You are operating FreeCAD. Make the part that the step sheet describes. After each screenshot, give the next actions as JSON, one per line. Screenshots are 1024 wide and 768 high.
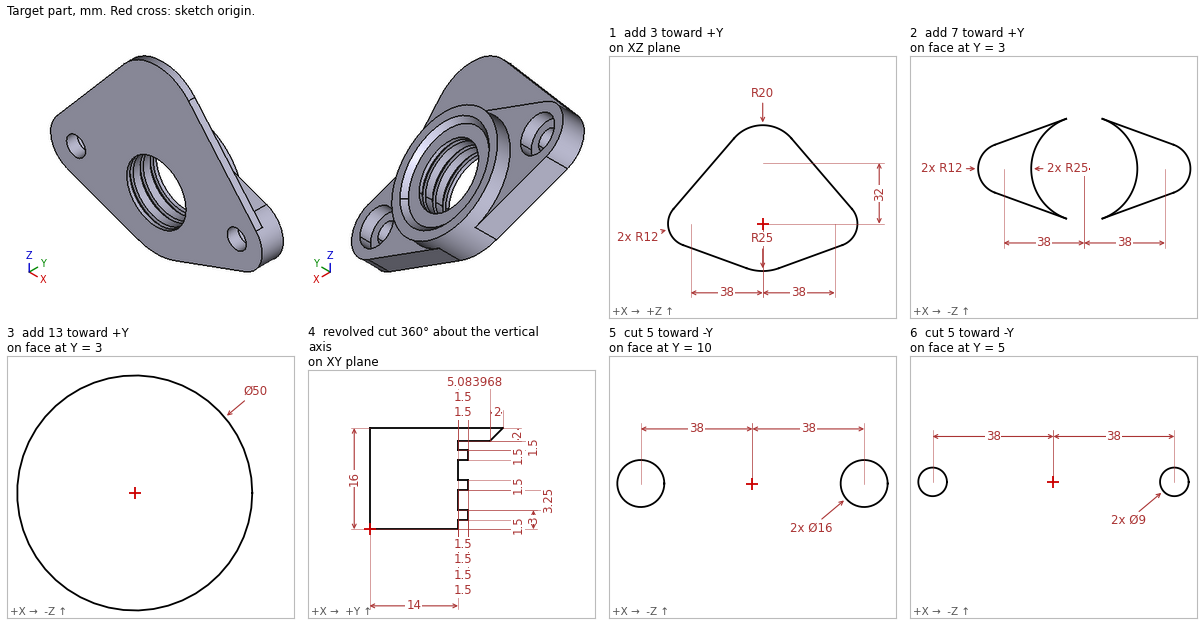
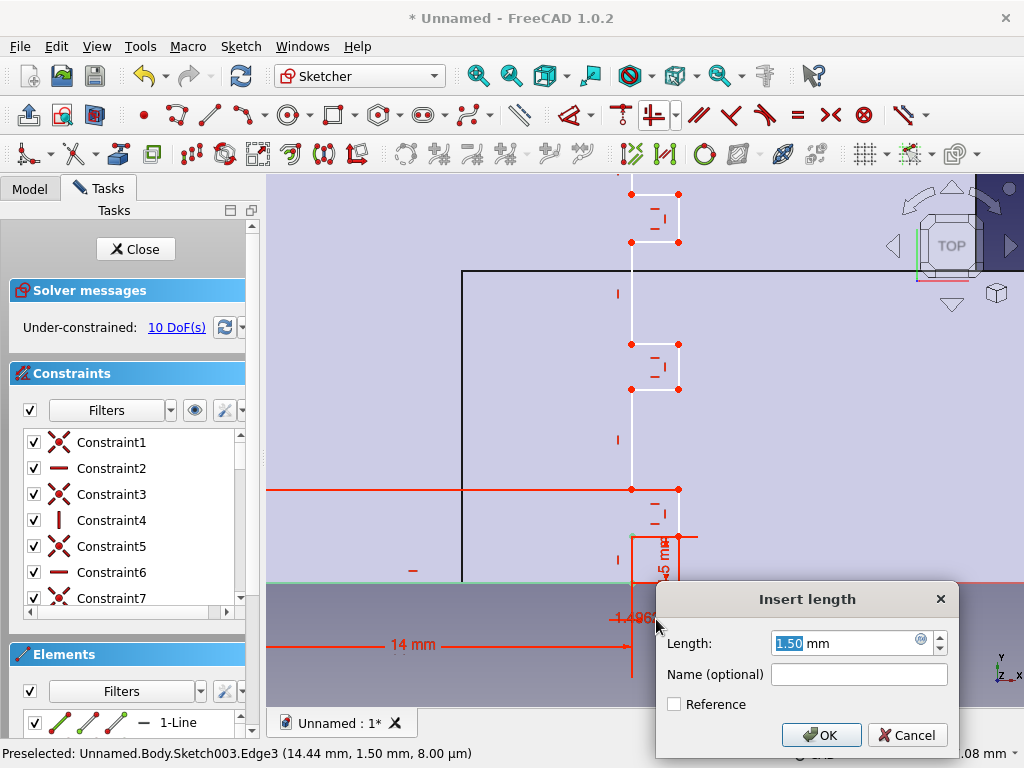
{"action": "type", "text": "1.5"}
{"action": "key", "text": "Return"}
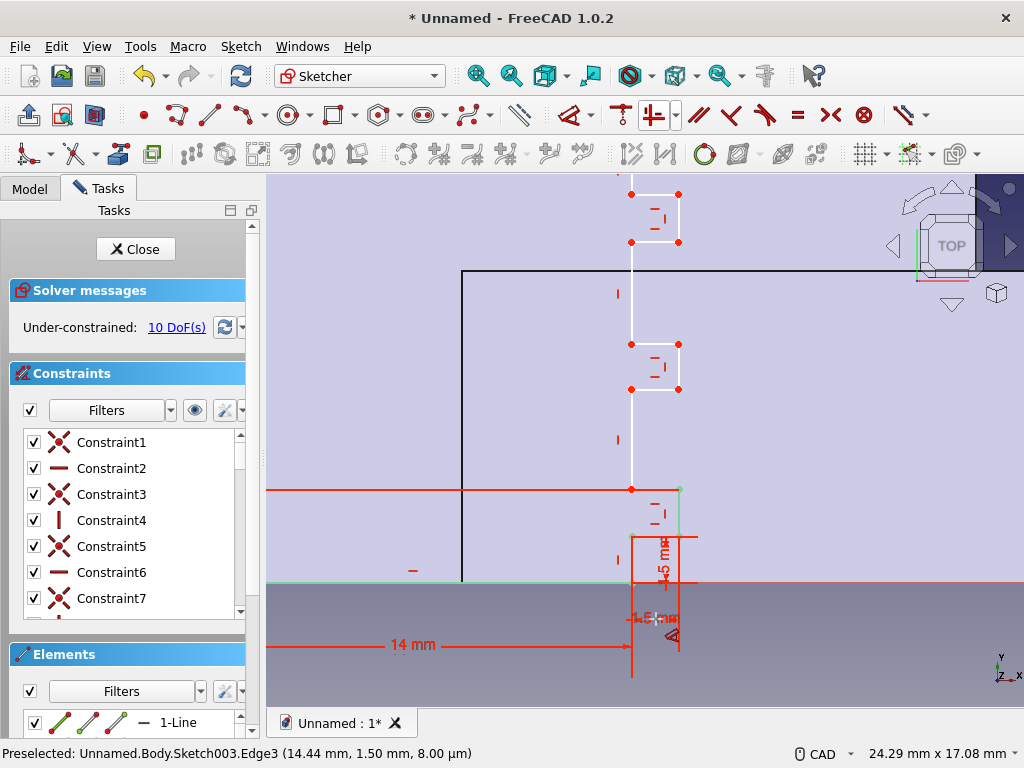
{"action": "left_click", "coordinate": [665, 490]}
{"action": "left_click", "coordinate": [655, 456]}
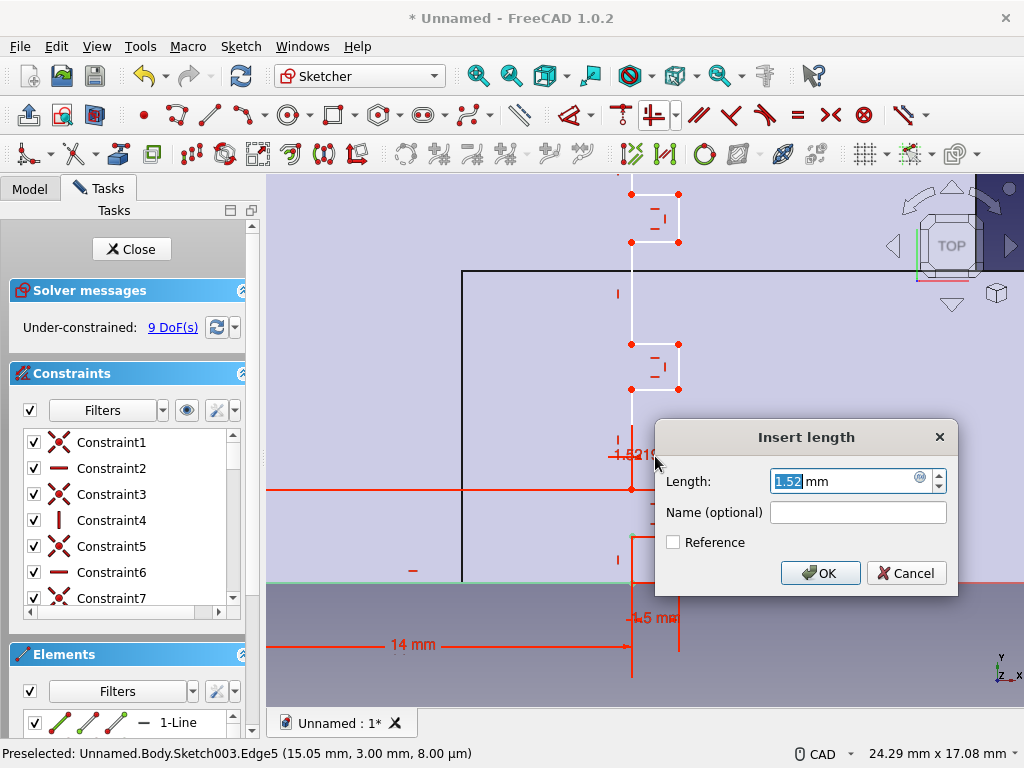
{"action": "type", "text": "1.5"}
{"action": "key", "text": "Return"}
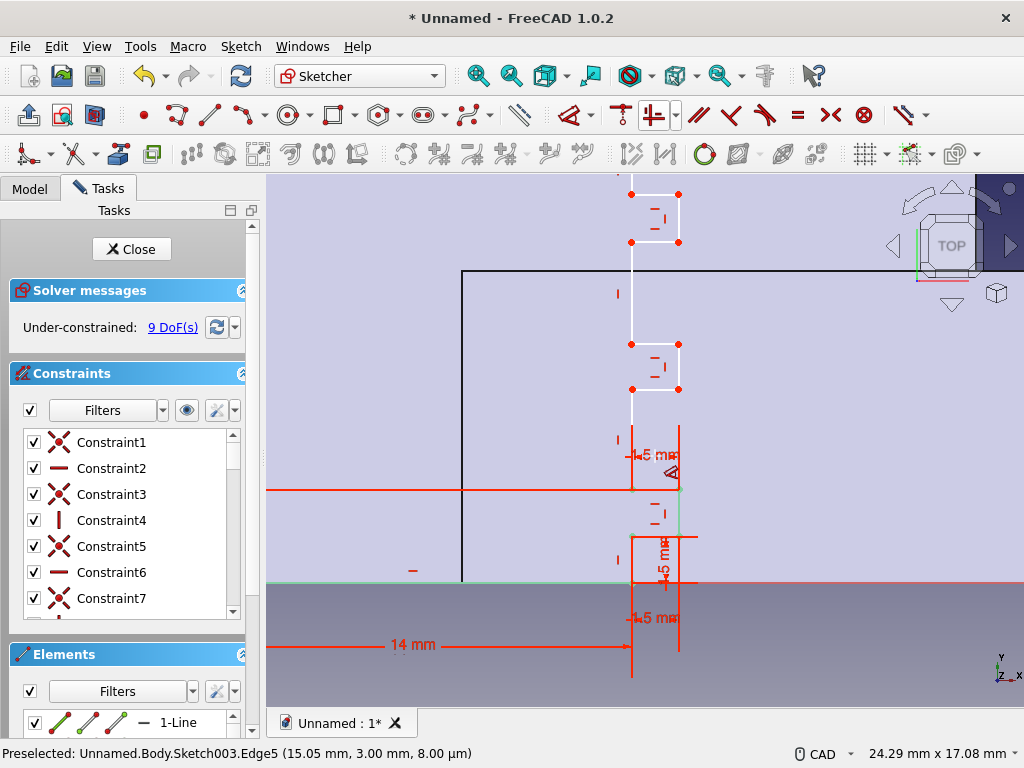
{"action": "left_click", "coordinate": [646, 390]}
{"action": "left_click", "coordinate": [656, 424]}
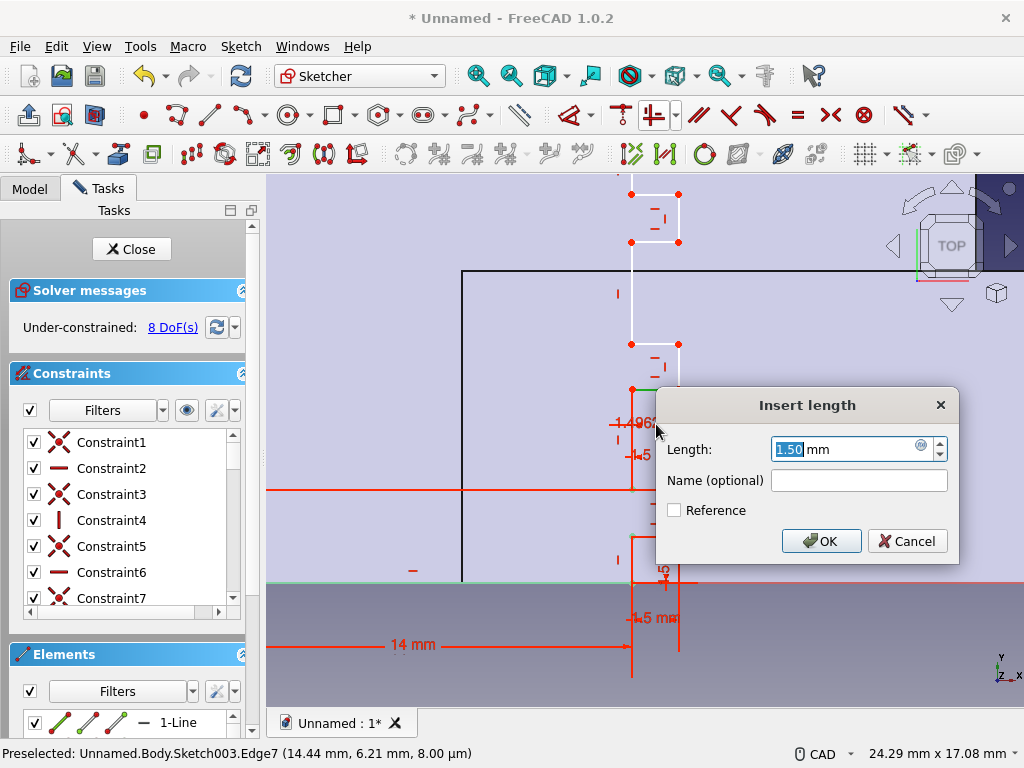
{"action": "type", "text": "1.5"}
{"action": "key", "text": "Return"}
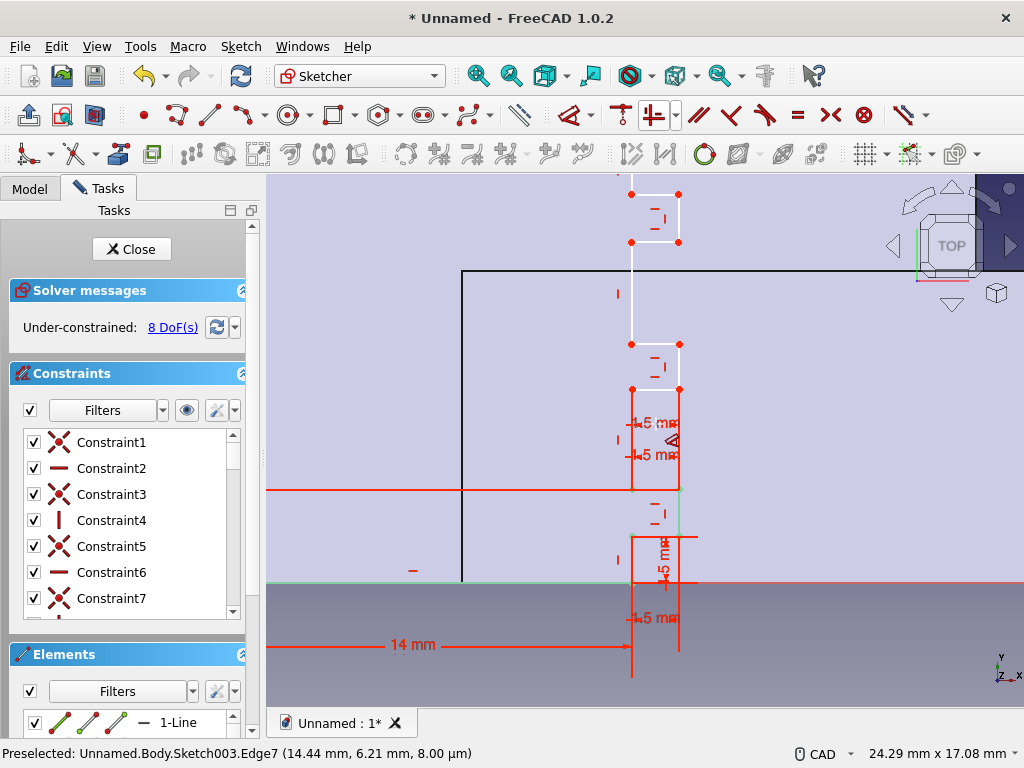
{"action": "left_click", "coordinate": [679, 376]}
{"action": "left_click", "coordinate": [713, 367]}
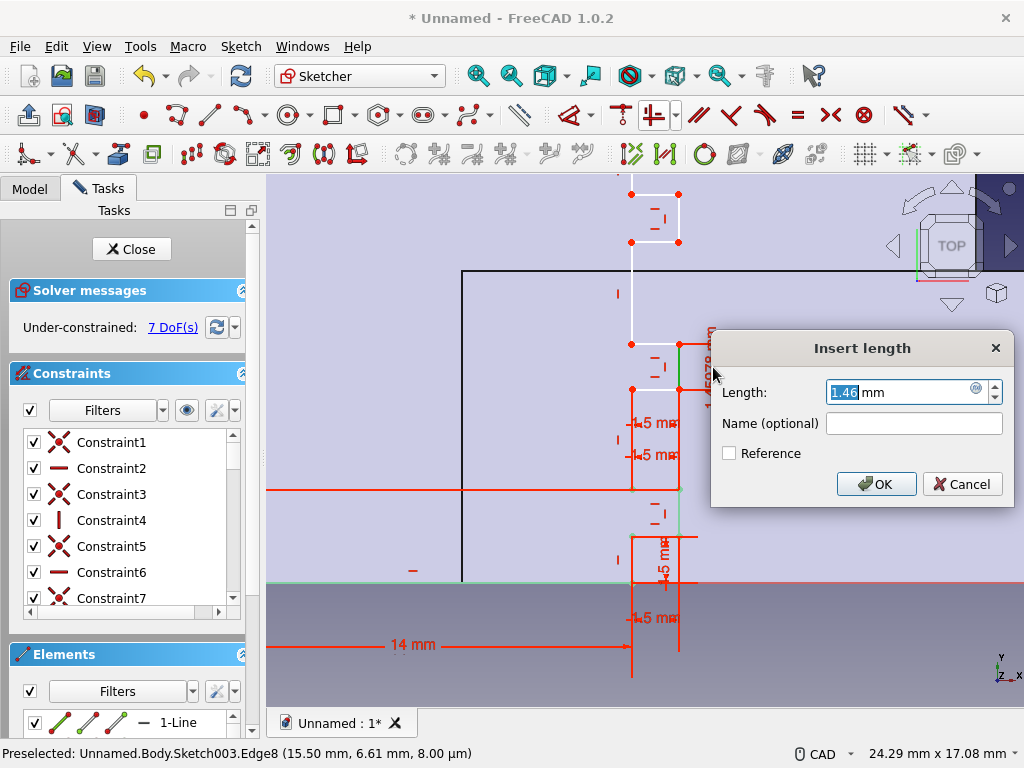
{"action": "type", "text": "1.5"}
{"action": "key", "text": "Return"}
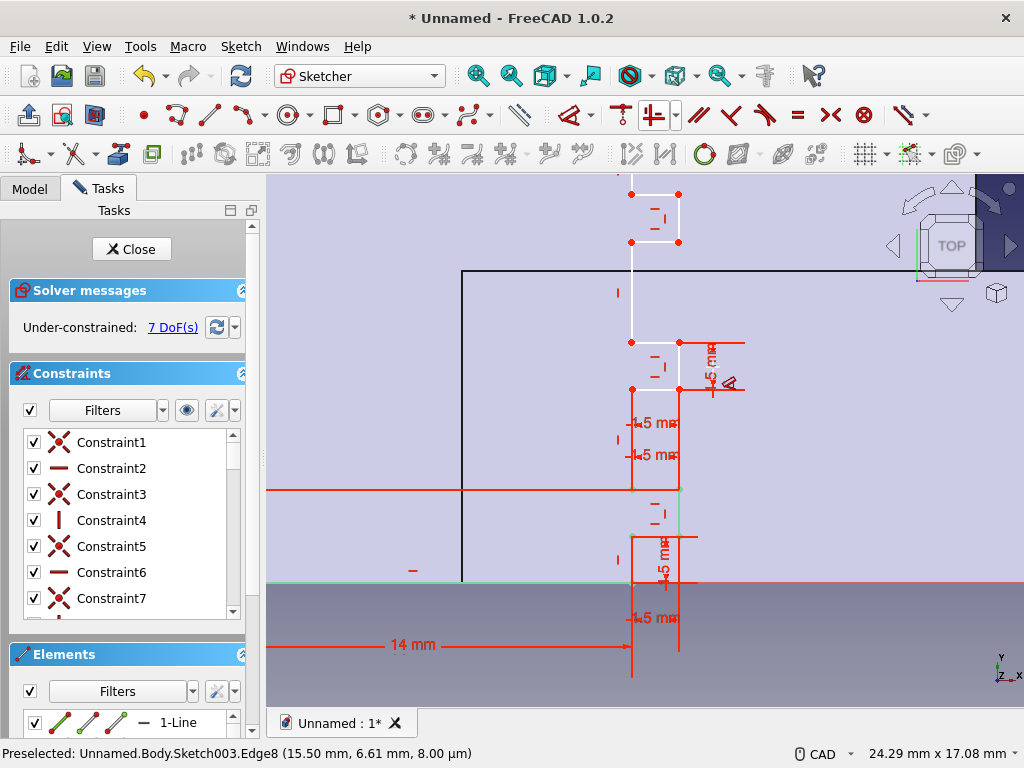
{"action": "left_click", "coordinate": [665, 343]}
{"action": "left_click", "coordinate": [655, 309]}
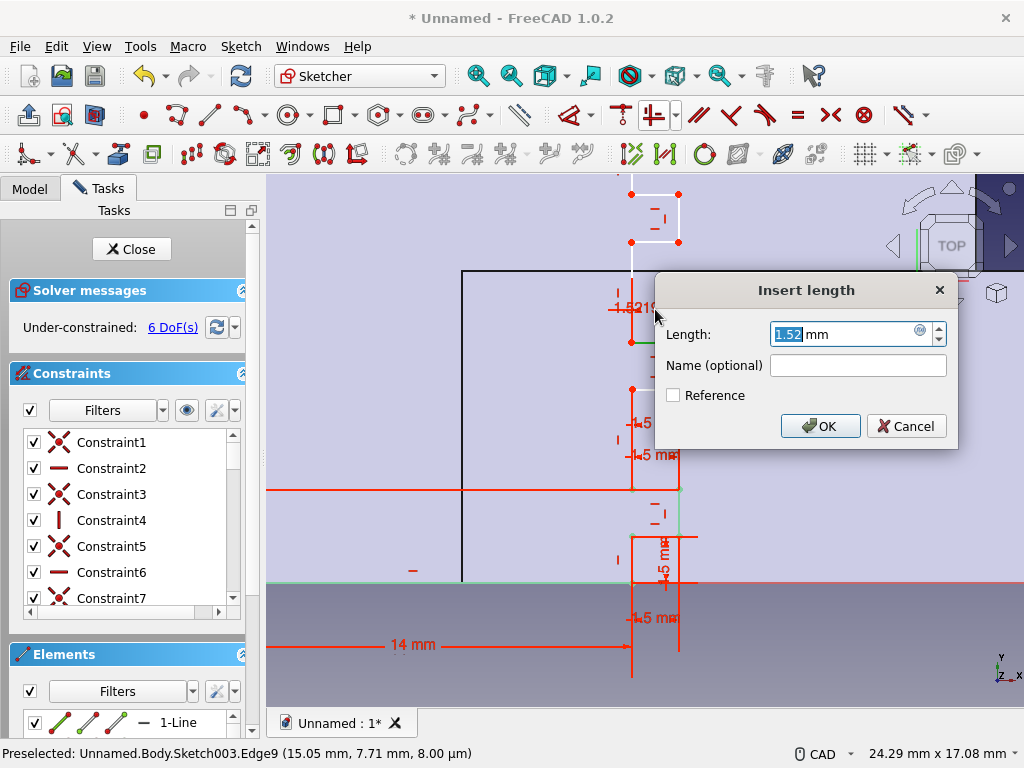
{"action": "type", "text": "1.5"}
{"action": "key", "text": "Return"}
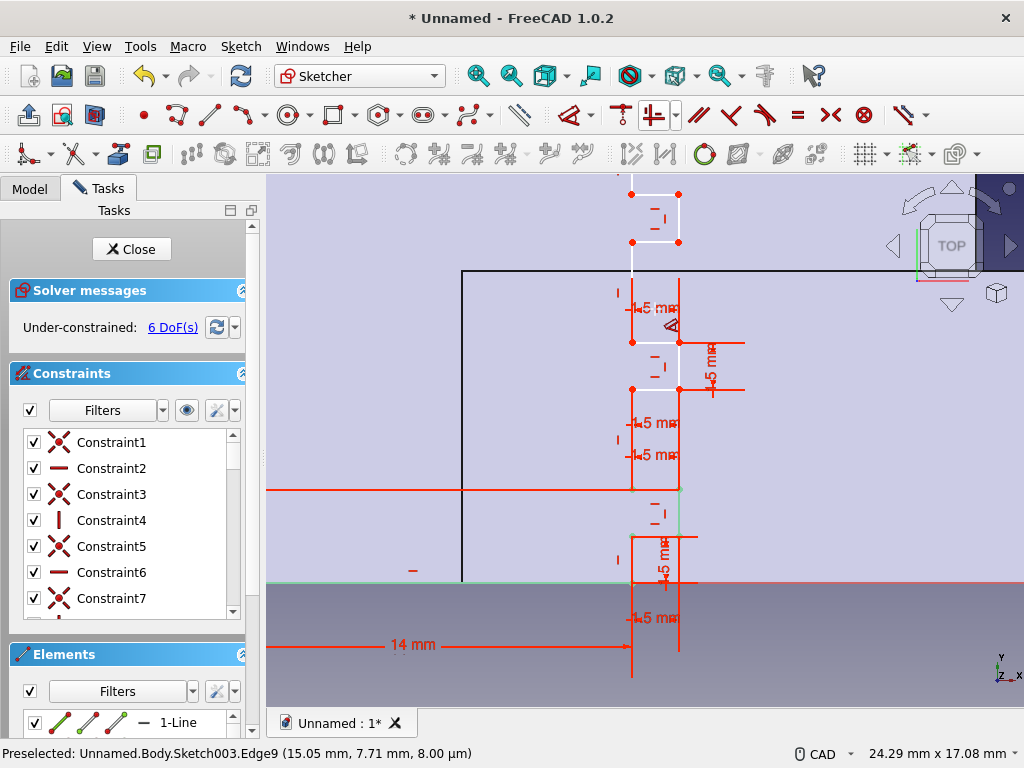
{"action": "left_click", "coordinate": [646, 242]}
{"action": "left_click", "coordinate": [656, 208]}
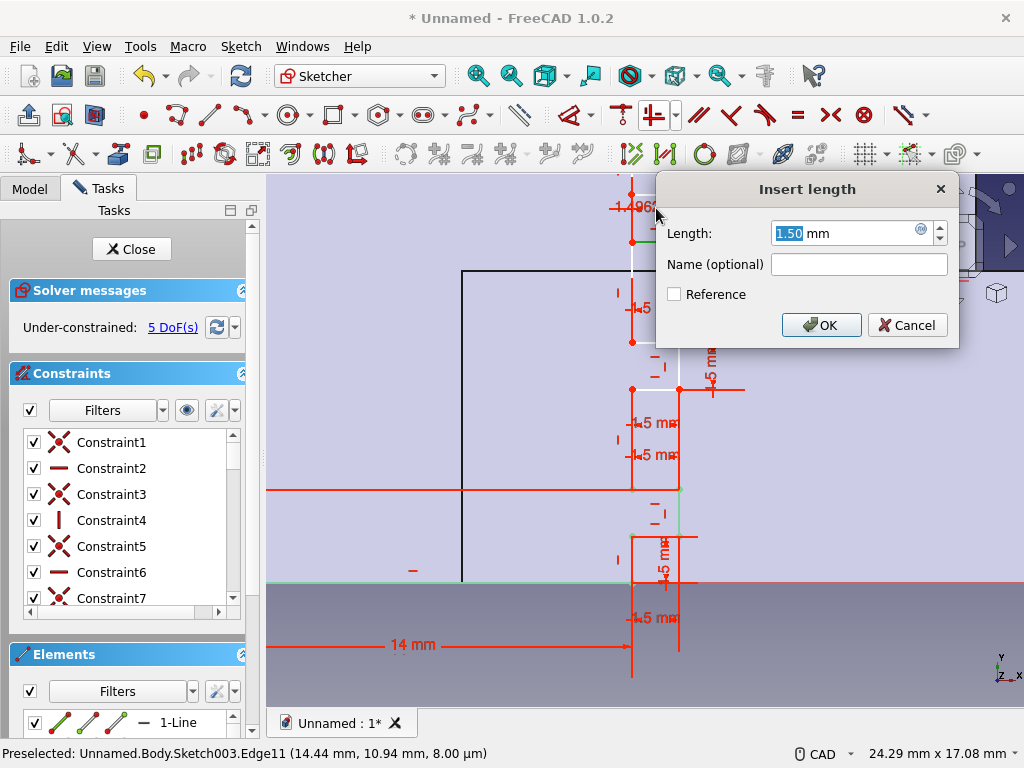
{"action": "type", "text": "1.5"}
{"action": "key", "text": "Return"}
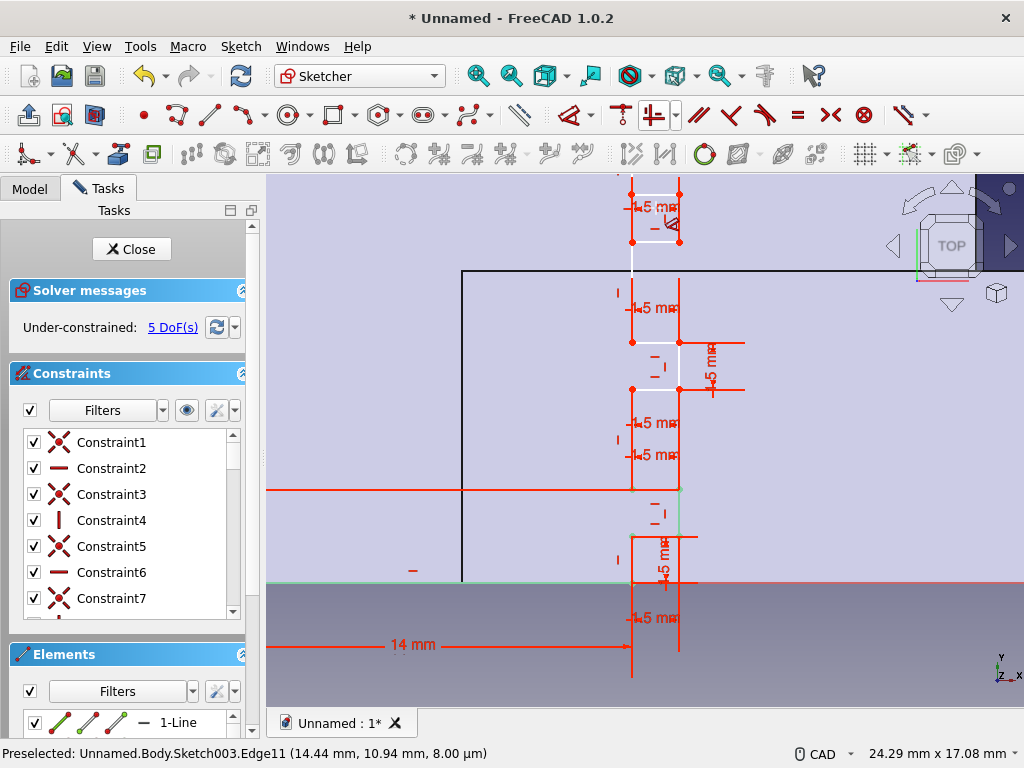
{"action": "left_click", "coordinate": [679, 228]}
{"action": "left_click", "coordinate": [713, 231]}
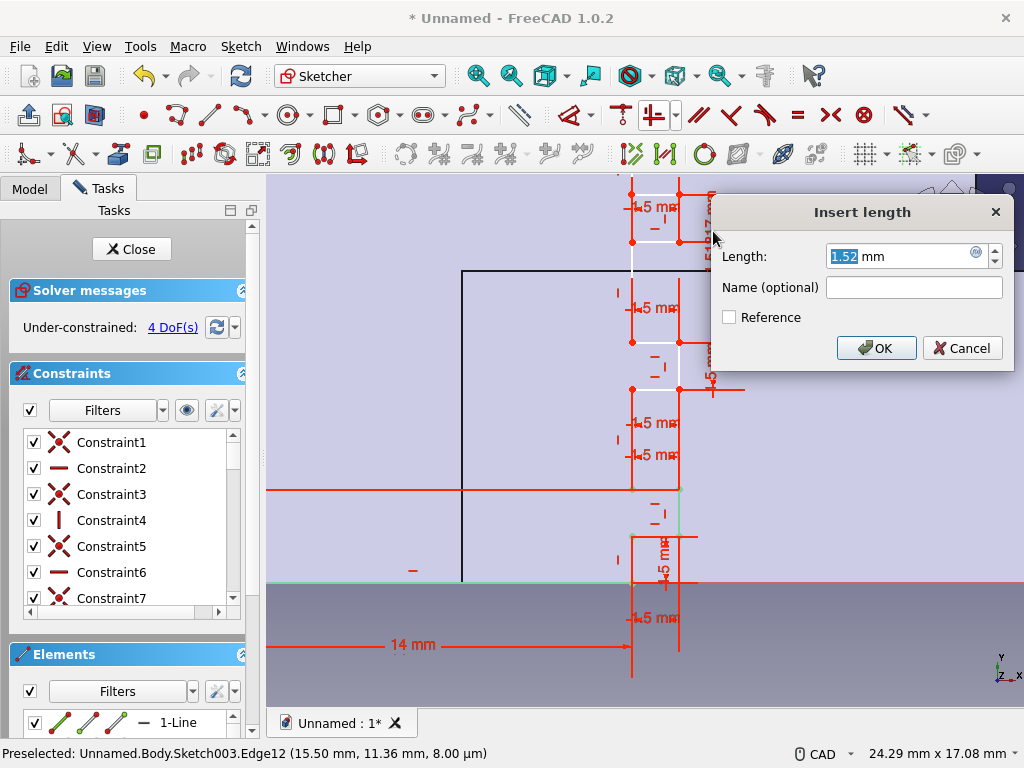
{"action": "type", "text": "1.5"}
{"action": "key", "text": "Return"}